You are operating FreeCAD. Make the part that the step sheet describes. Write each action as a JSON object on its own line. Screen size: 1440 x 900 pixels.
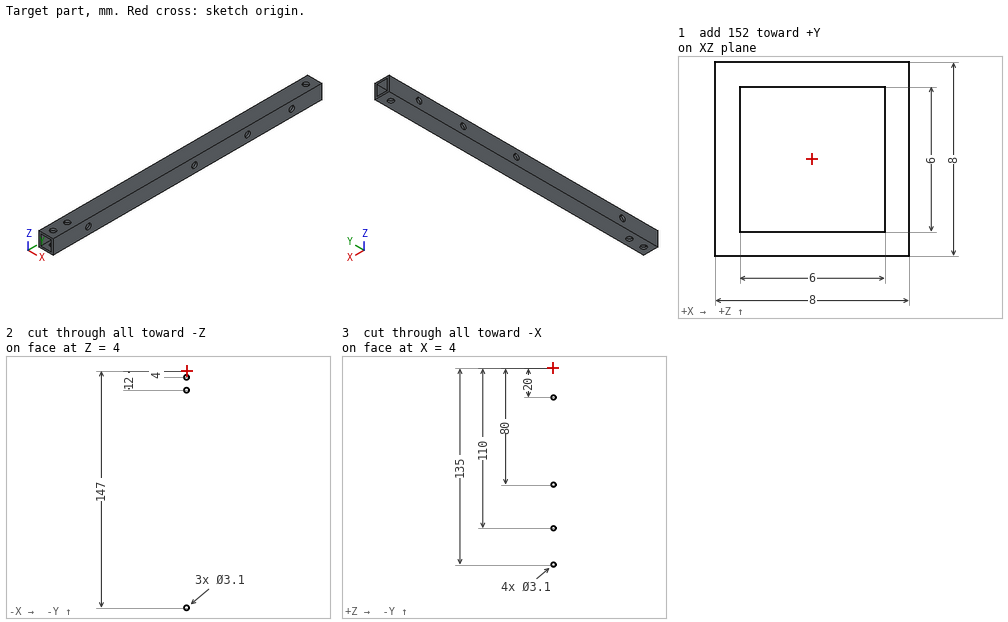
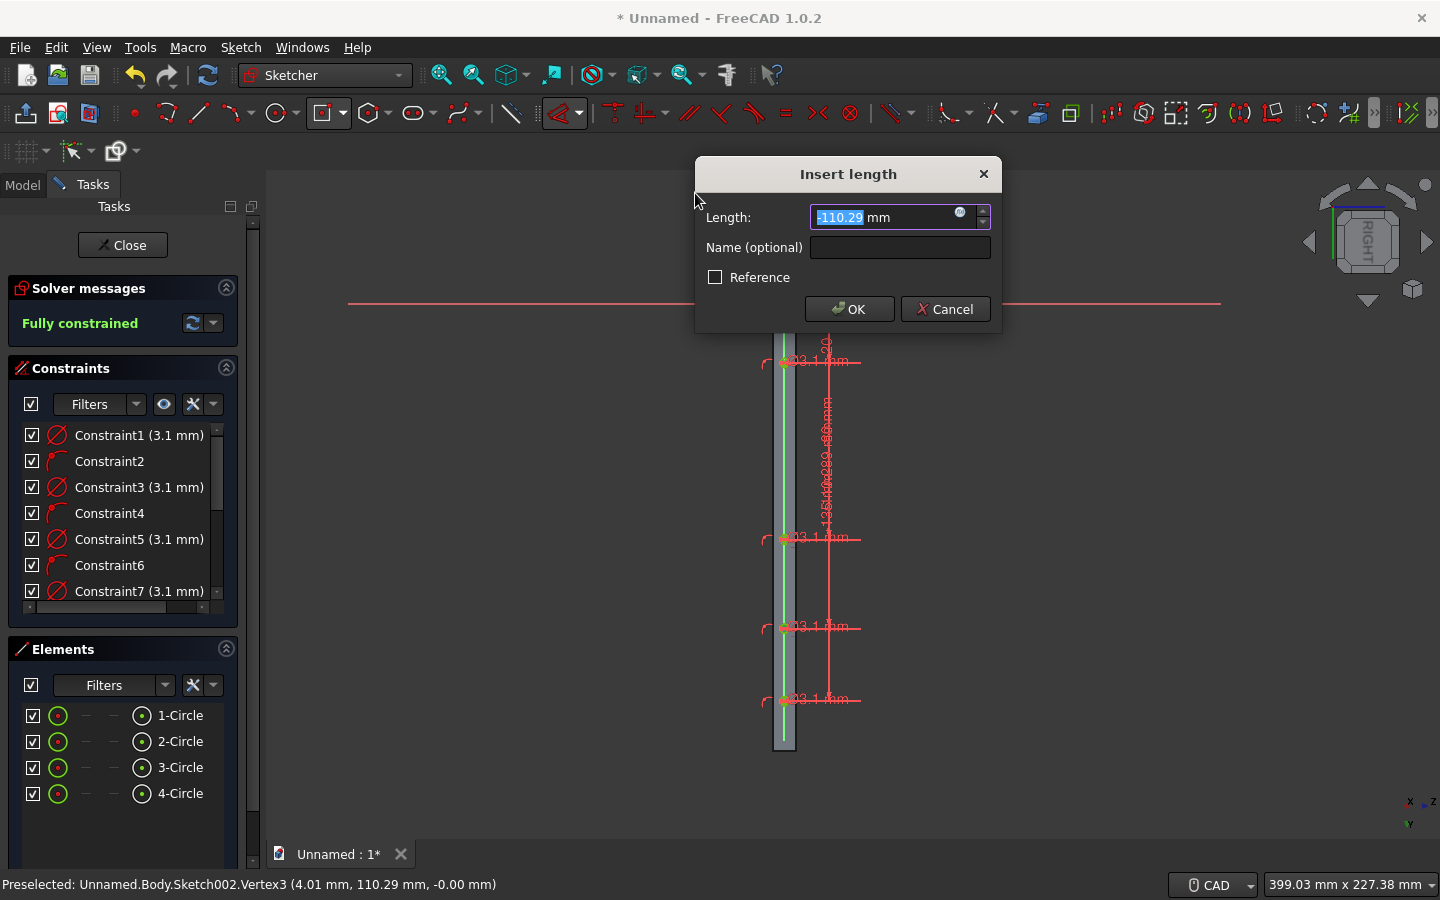
{"action": "type", "text": "-110"}
{"action": "key", "text": "Return"}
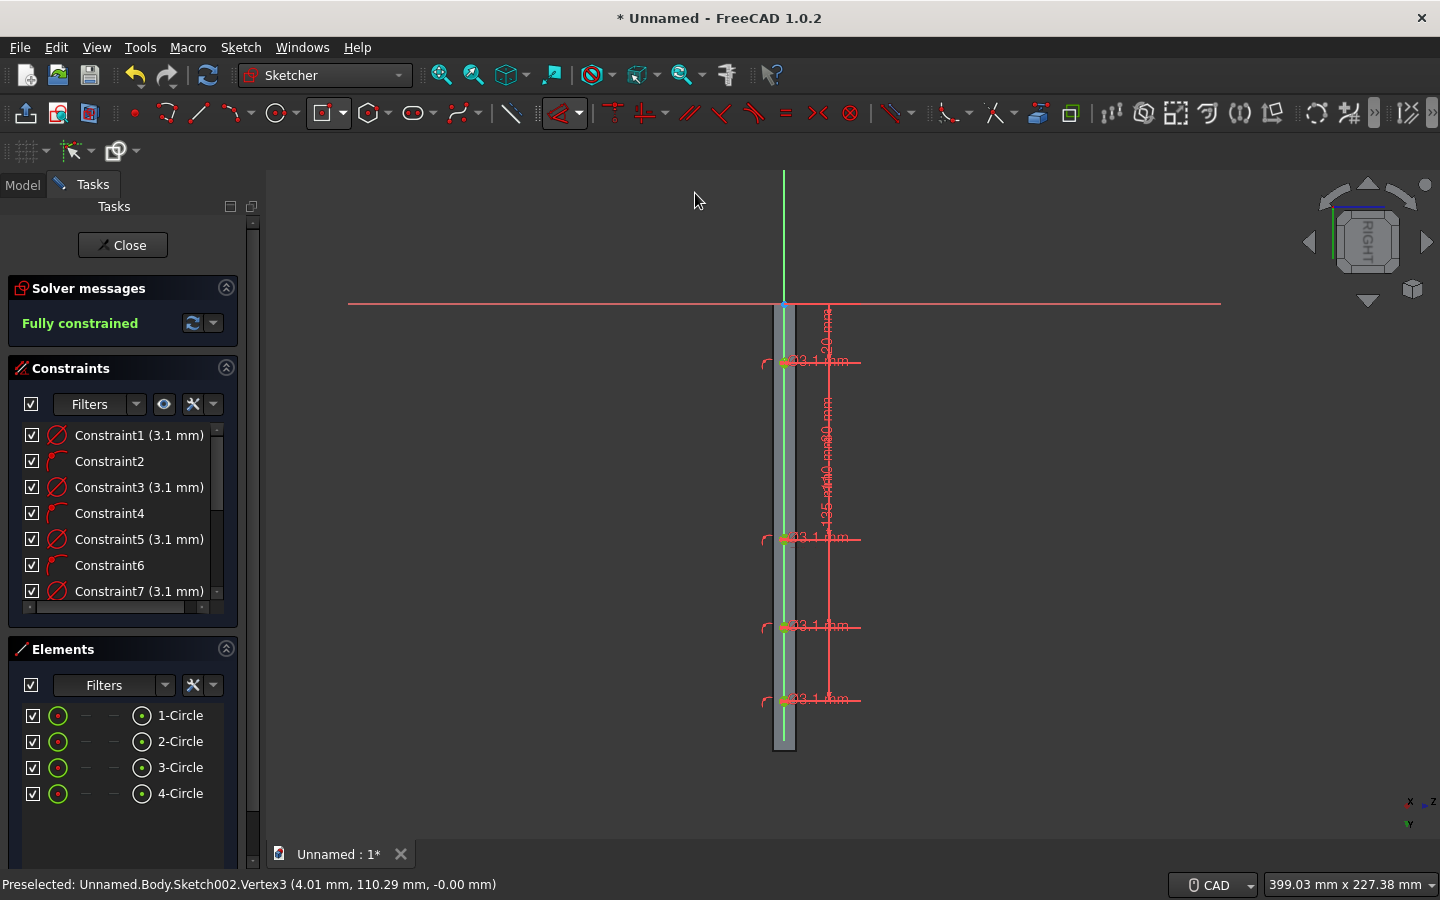
{"action": "left_click", "coordinate": [123, 245]}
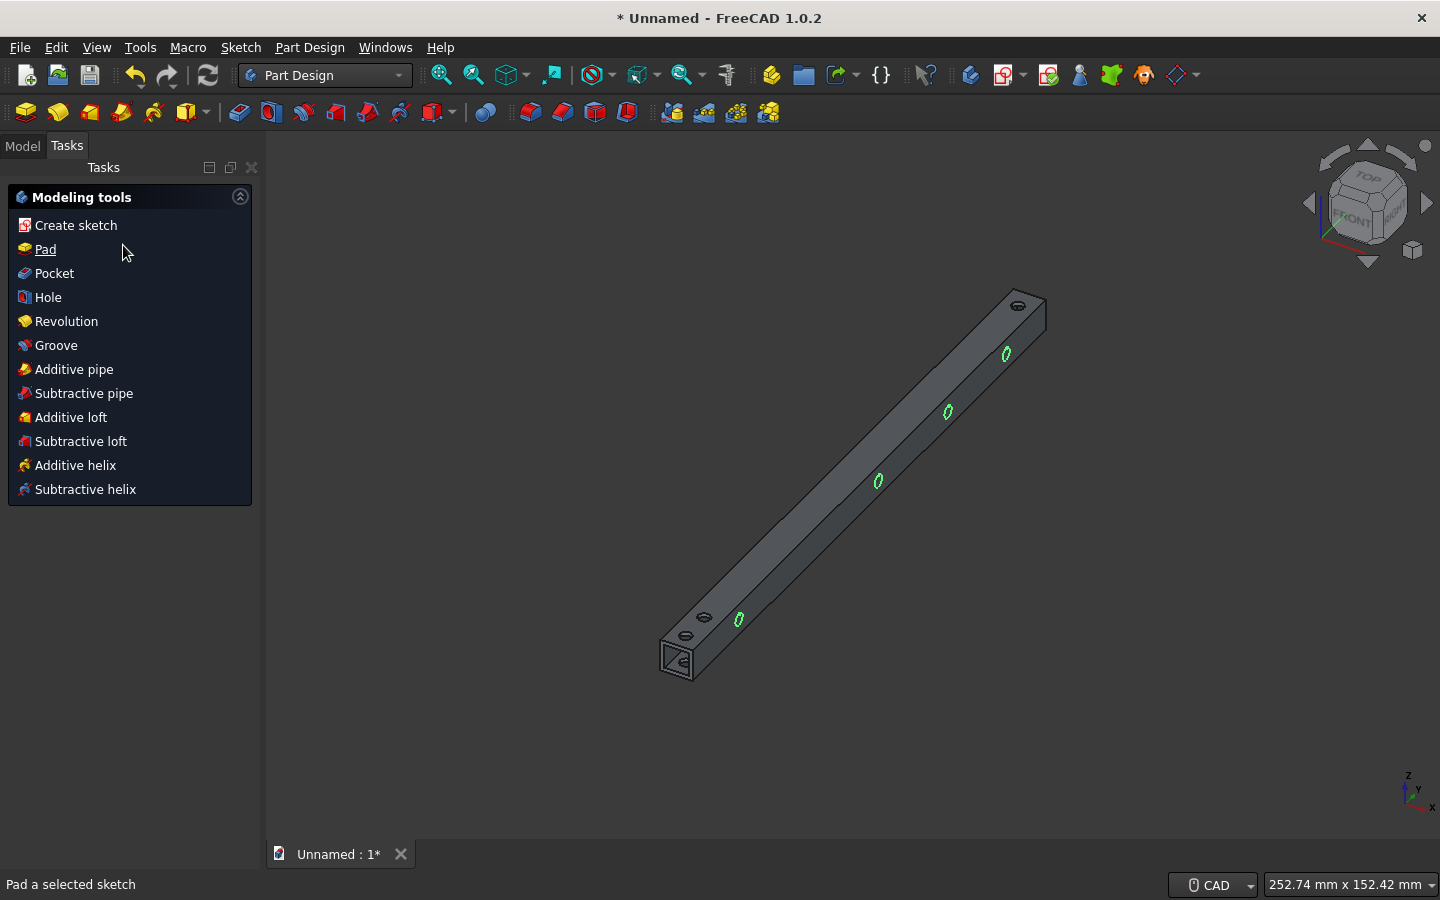
{"action": "left_click", "coordinate": [240, 112]}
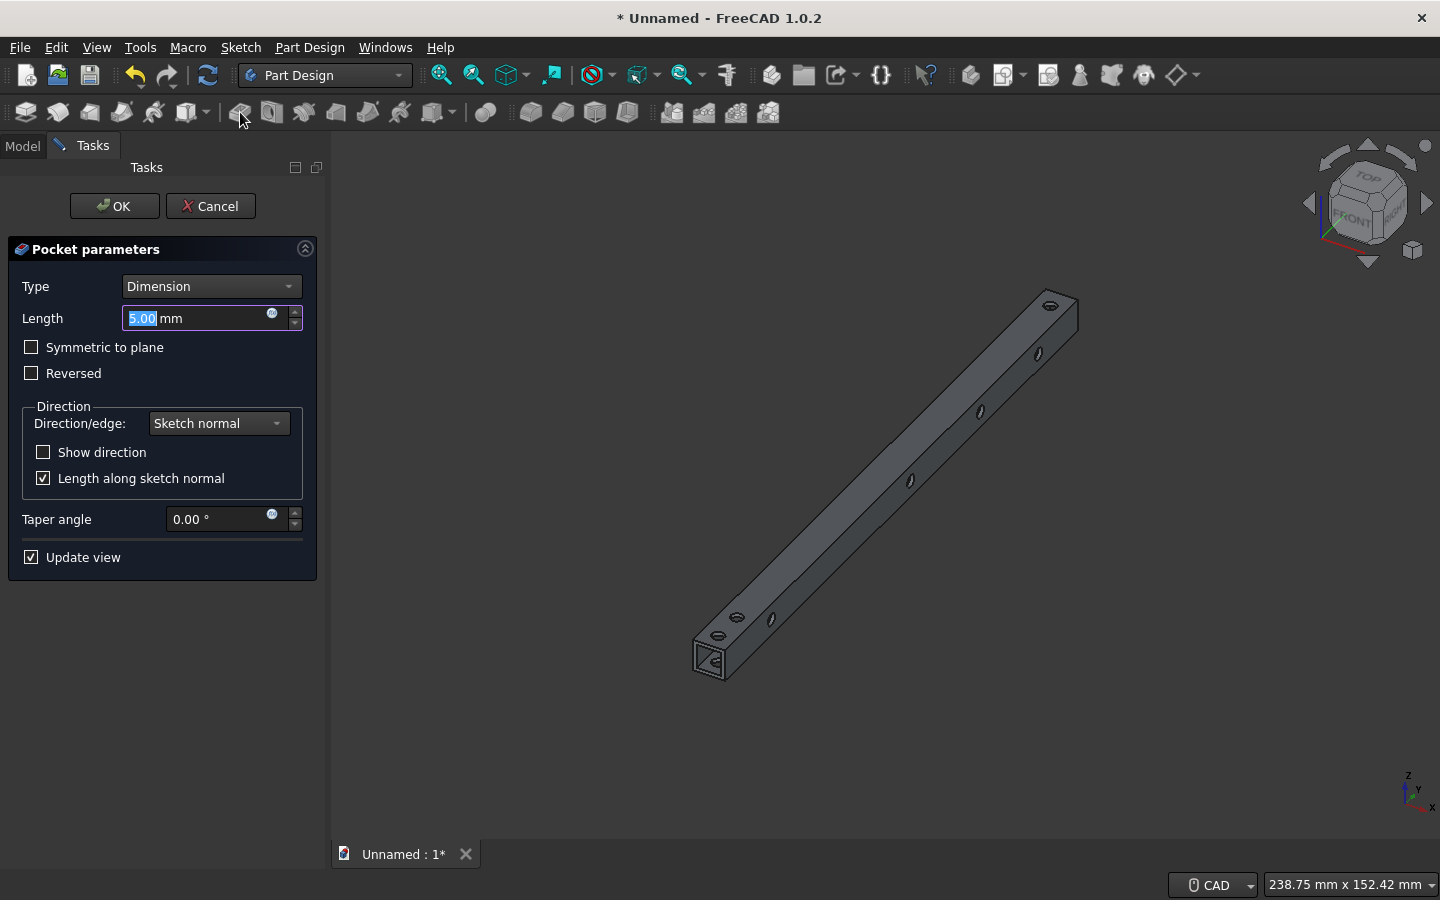
{"action": "left_click", "coordinate": [212, 286]}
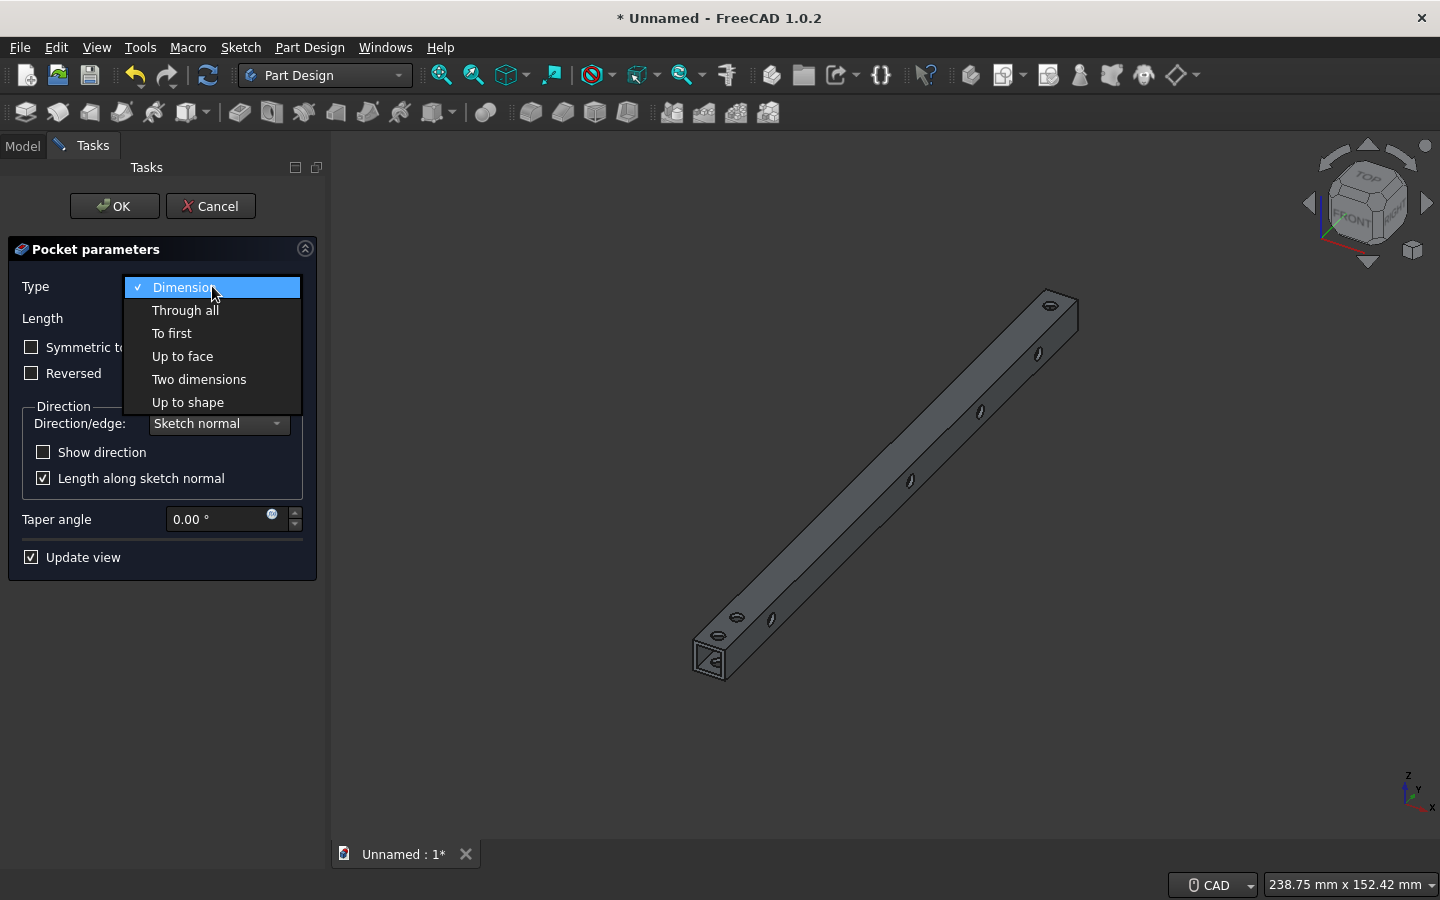
{"action": "left_click", "coordinate": [212, 310]}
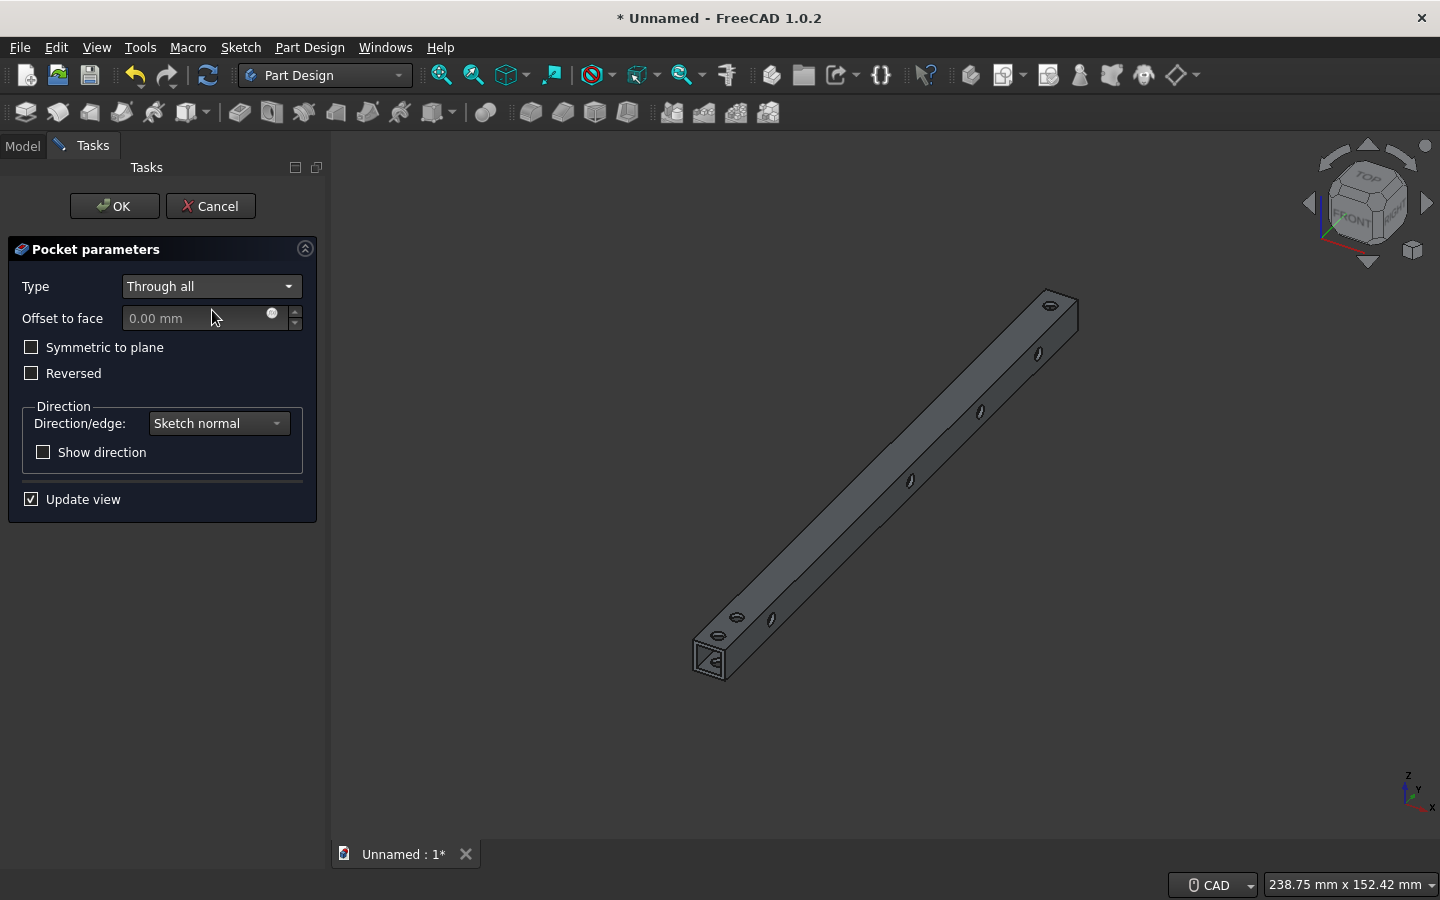
{"action": "left_click", "coordinate": [115, 206]}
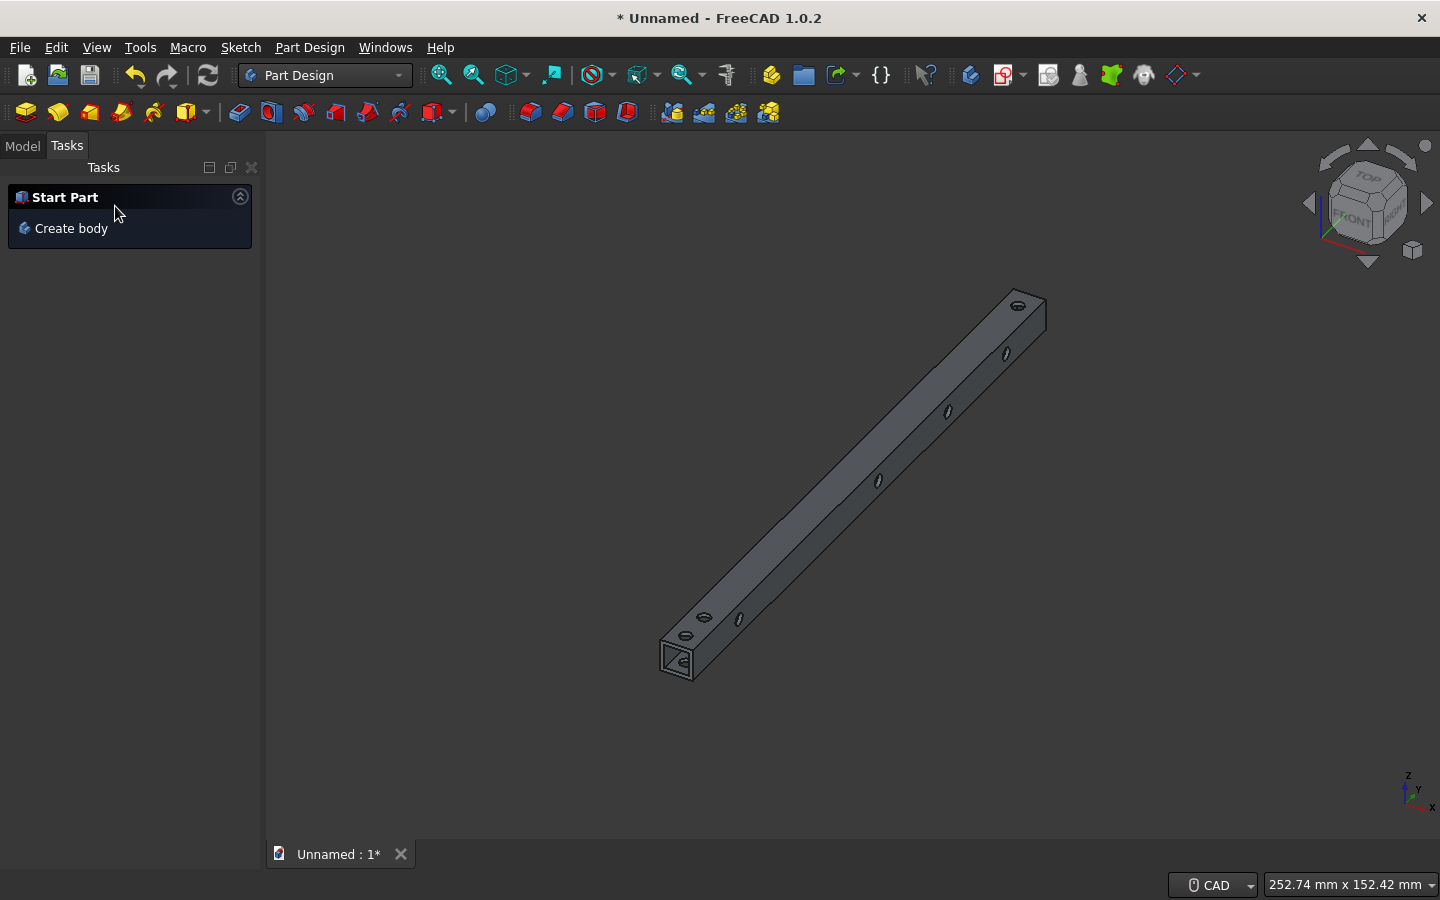
{"action": "key", "text": "0"}